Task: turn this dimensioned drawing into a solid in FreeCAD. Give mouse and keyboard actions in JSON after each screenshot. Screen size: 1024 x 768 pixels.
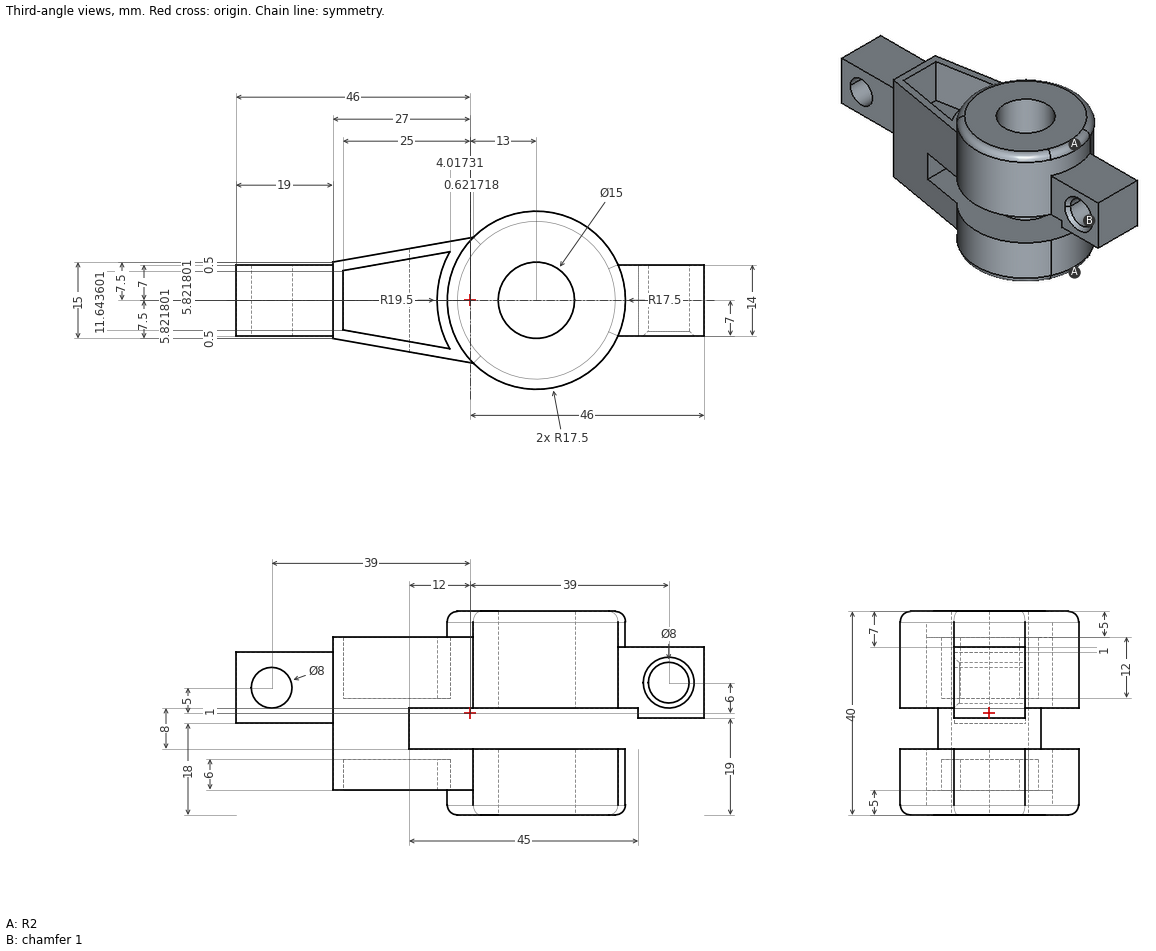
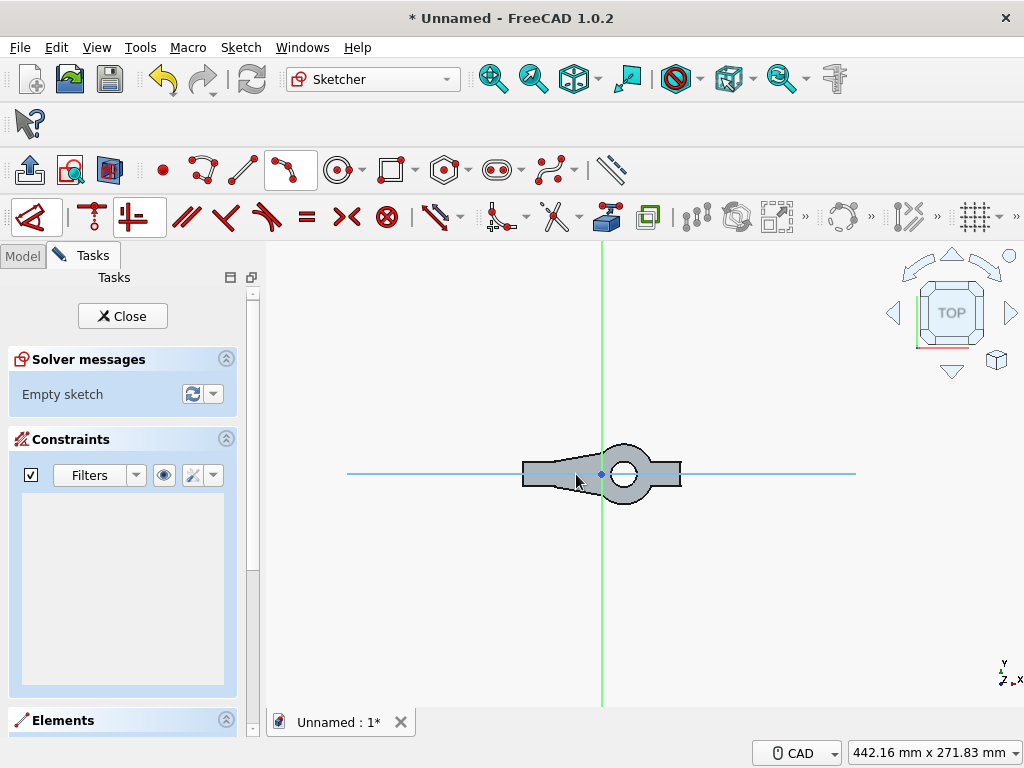
{"action": "scroll", "coordinate": [675, 474], "scroll_direction": "up", "scroll_amount": 12}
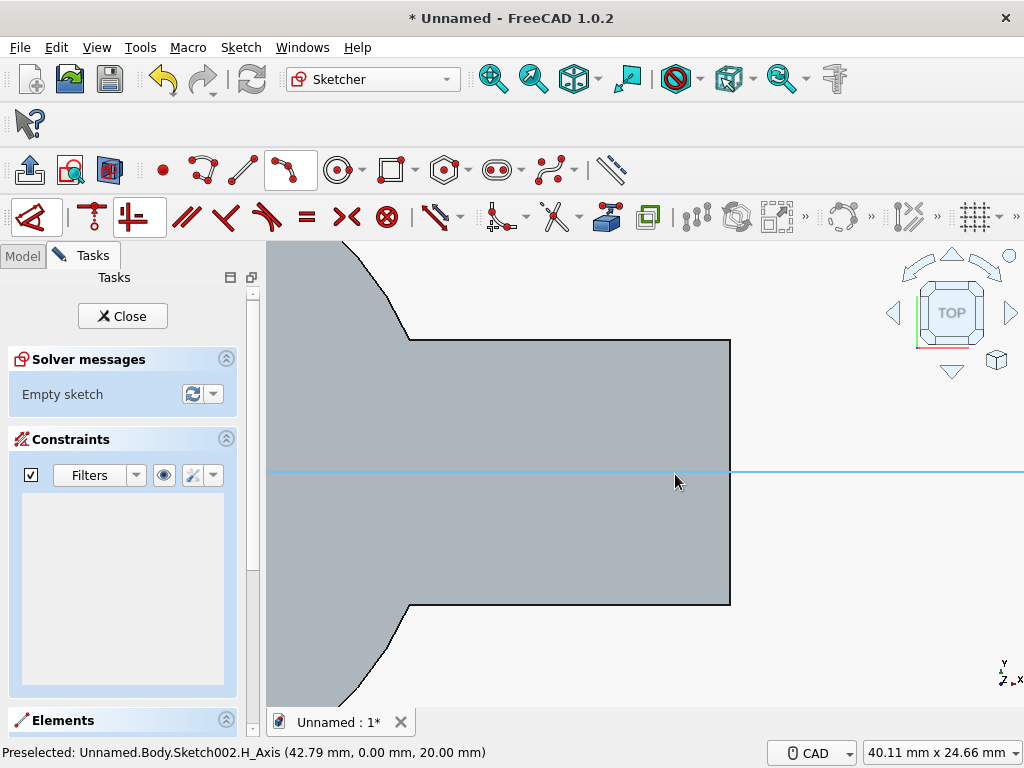
{"action": "left_click", "coordinate": [204, 170]}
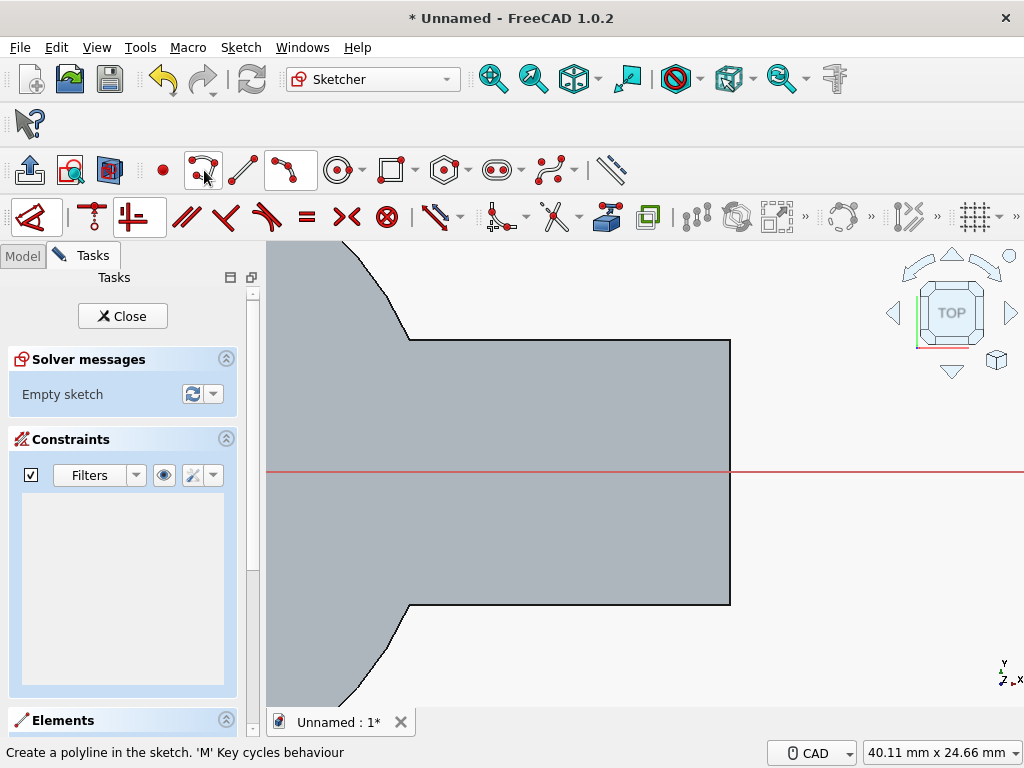
{"action": "left_click", "coordinate": [410, 605]}
{"action": "left_click", "coordinate": [730, 605]}
{"action": "left_click", "coordinate": [730, 340]}
{"action": "left_click", "coordinate": [410, 340]}
{"action": "right_click", "coordinate": [410, 340]}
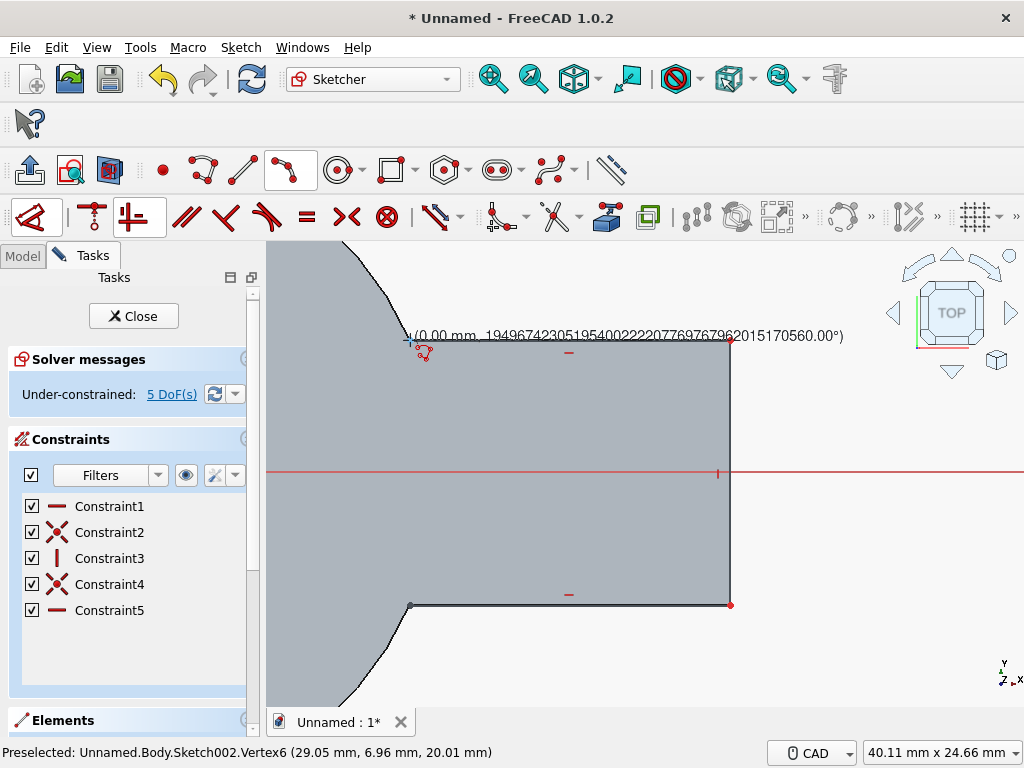
{"action": "left_click", "coordinate": [284, 170]}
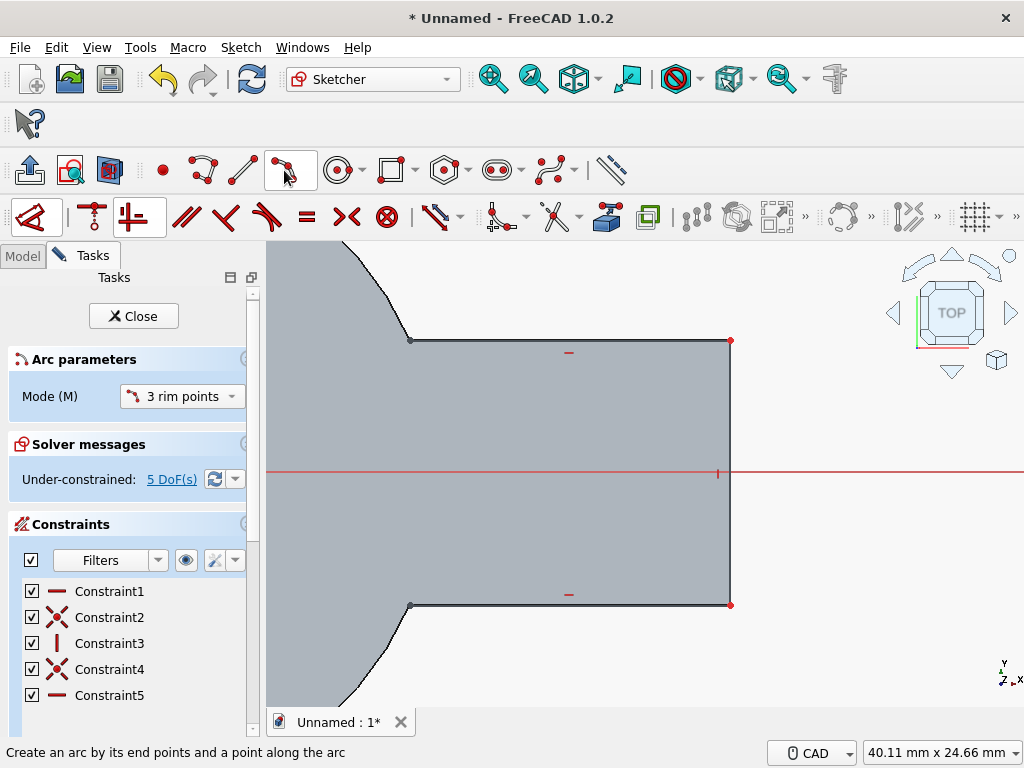
{"action": "left_click", "coordinate": [410, 341]}
{"action": "left_click", "coordinate": [410, 606]}
{"action": "left_click", "coordinate": [436, 500]}
{"action": "key", "text": "Escape"}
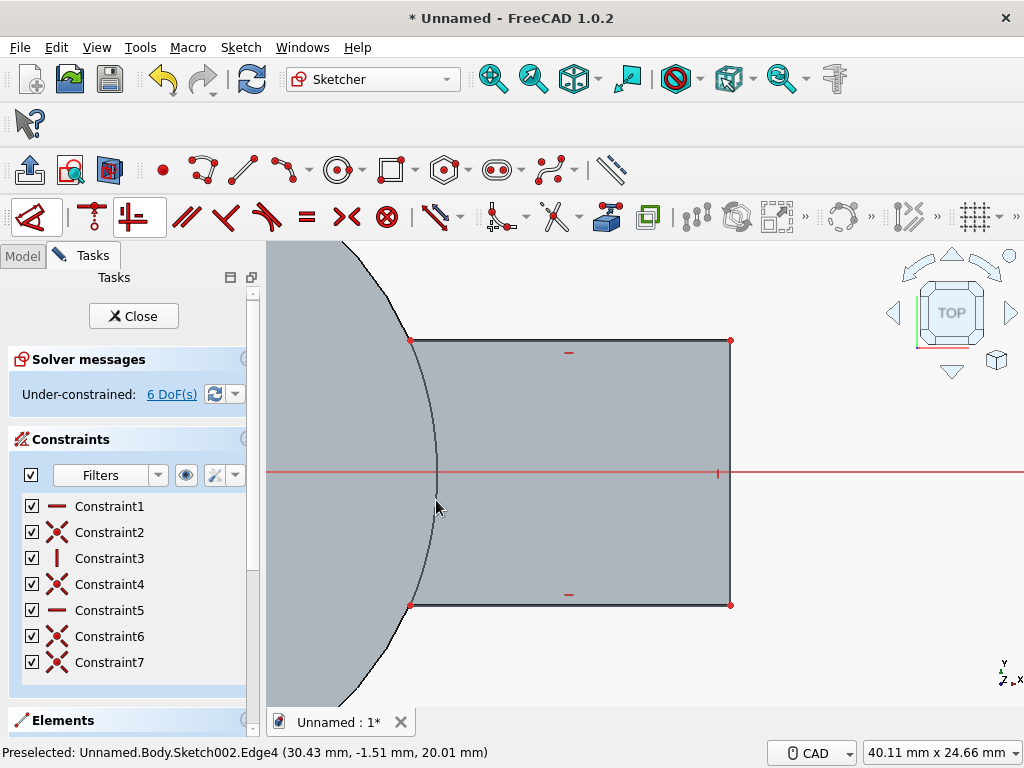
{"action": "scroll", "coordinate": [859, 477], "scroll_direction": "down", "scroll_amount": 2}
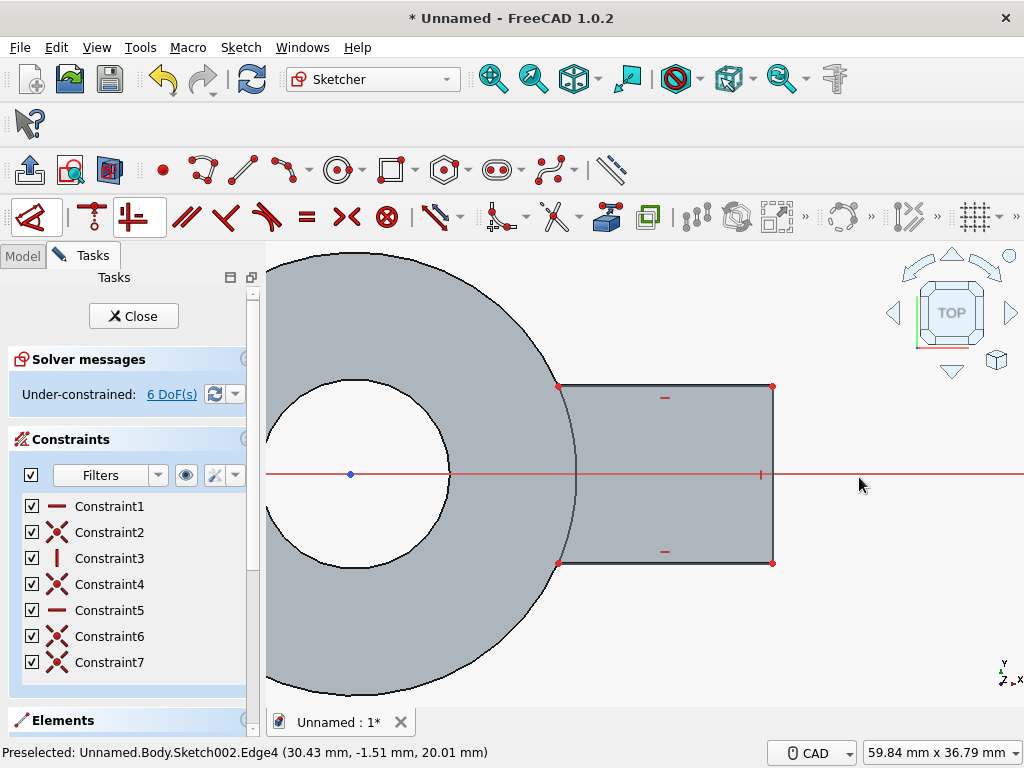
{"action": "left_click", "coordinate": [350, 475]}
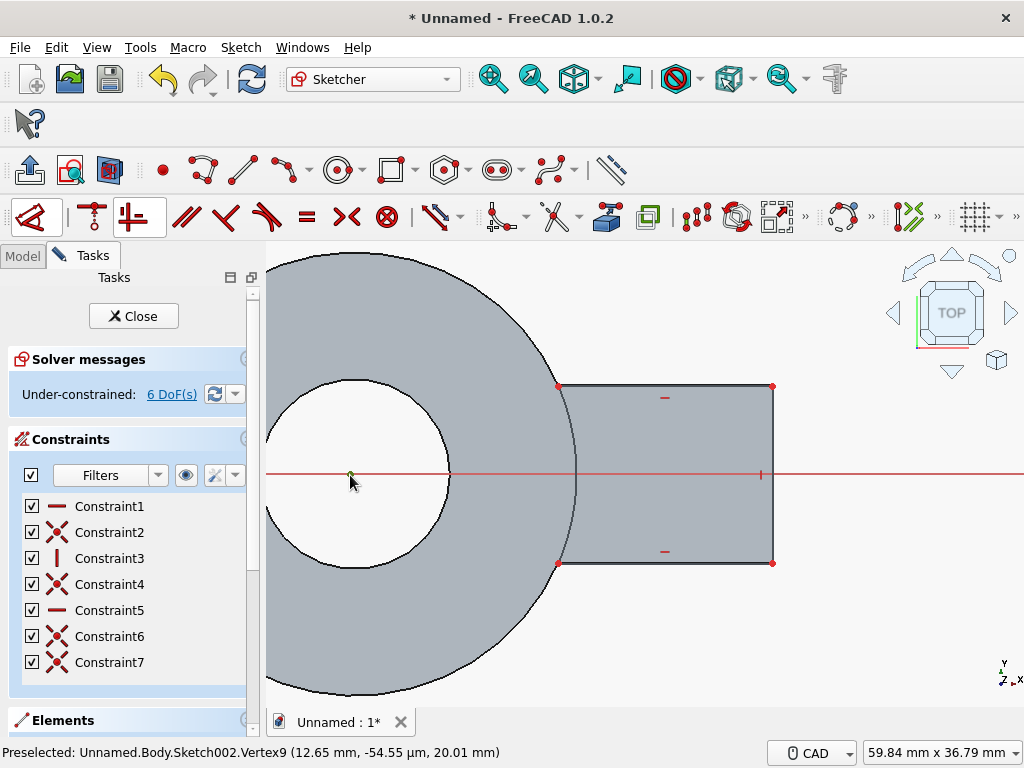
{"action": "left_click", "coordinate": [334, 474]}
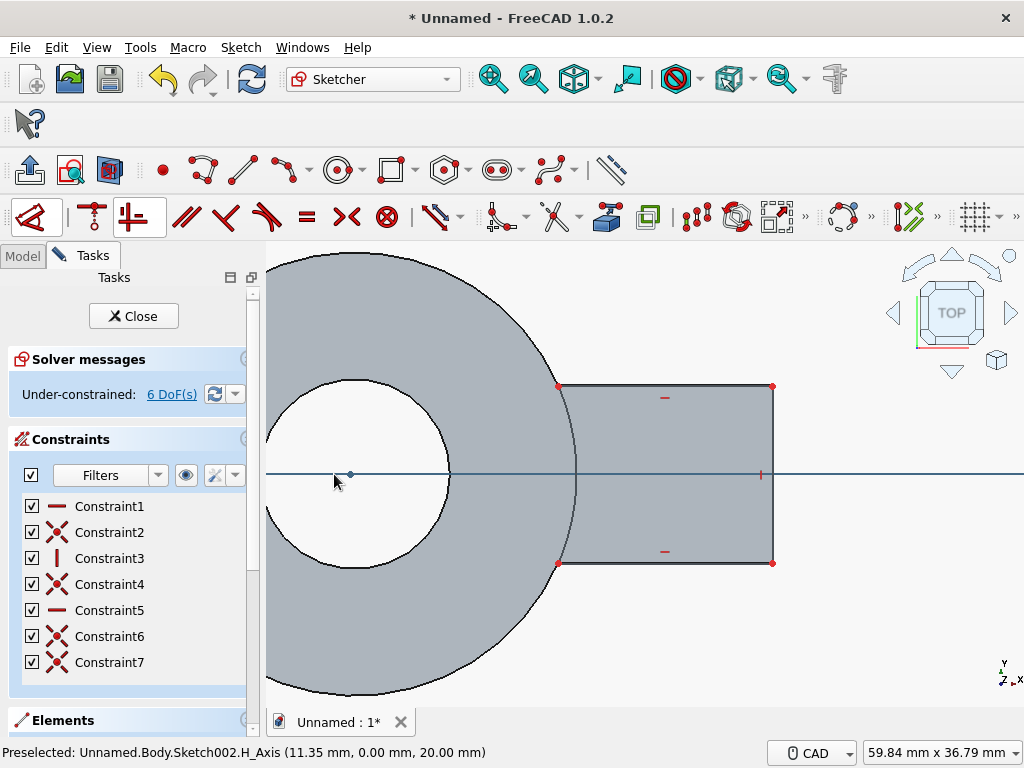
{"action": "left_click", "coordinate": [92, 218]}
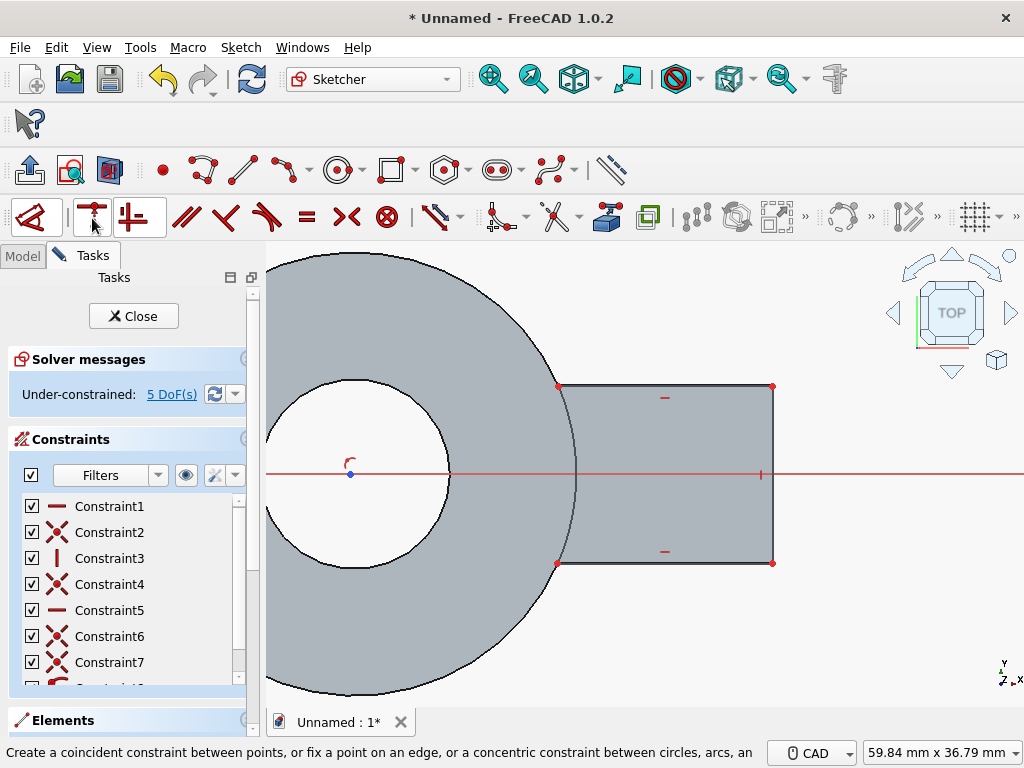
{"action": "left_click", "coordinate": [573, 511]}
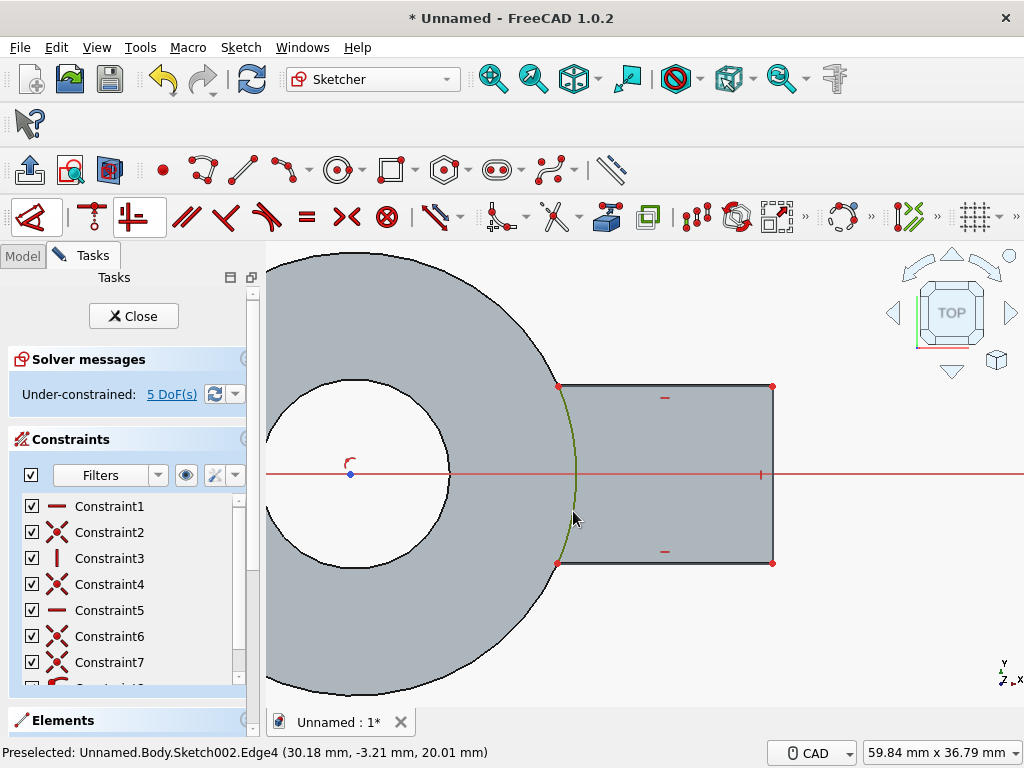
{"action": "key", "text": "k r"}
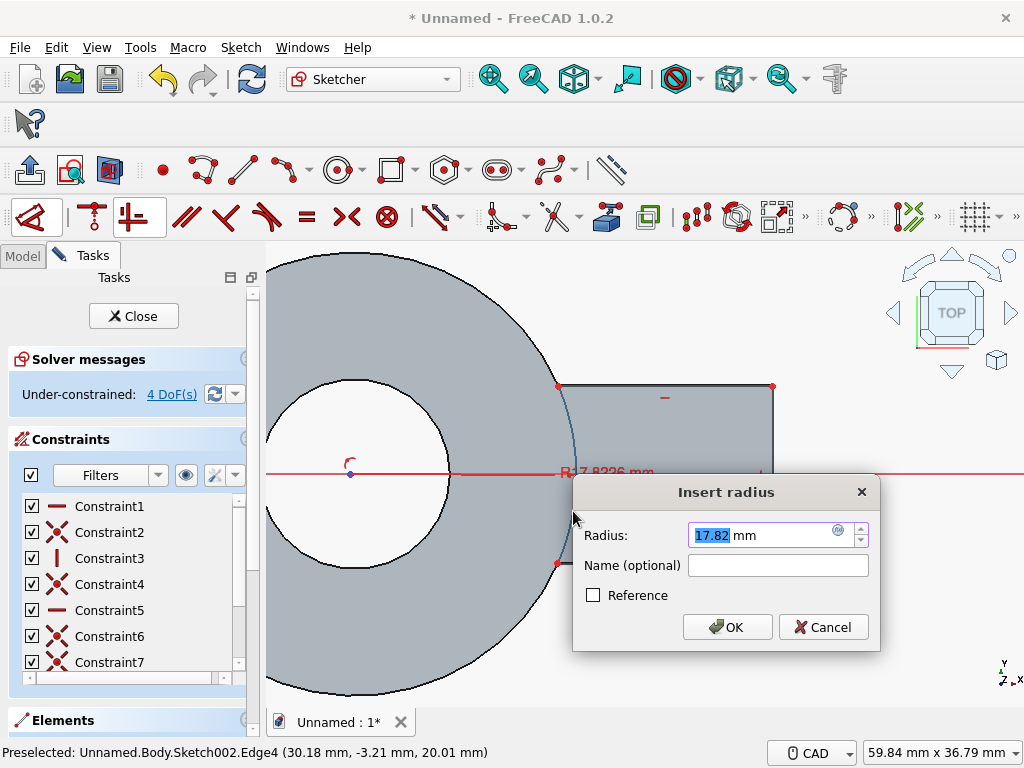
{"action": "type", "text": "17.5"}
{"action": "key", "text": "Return"}